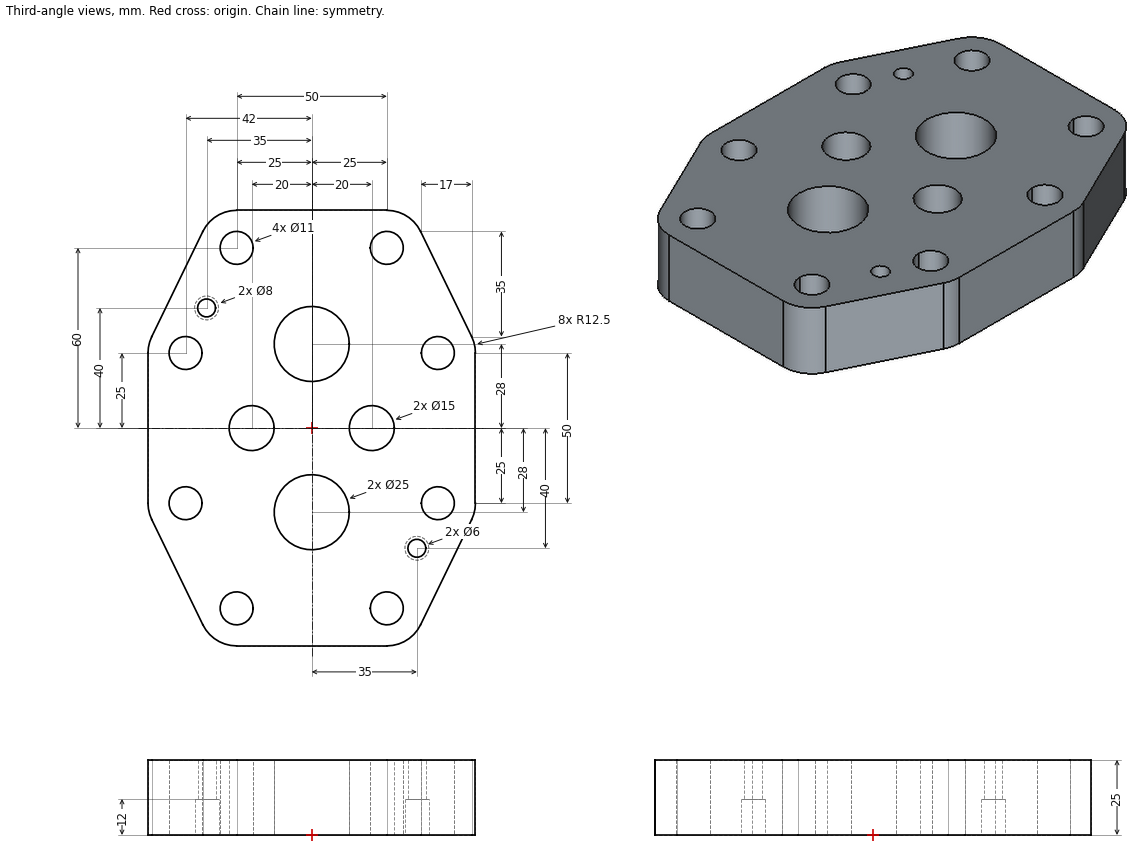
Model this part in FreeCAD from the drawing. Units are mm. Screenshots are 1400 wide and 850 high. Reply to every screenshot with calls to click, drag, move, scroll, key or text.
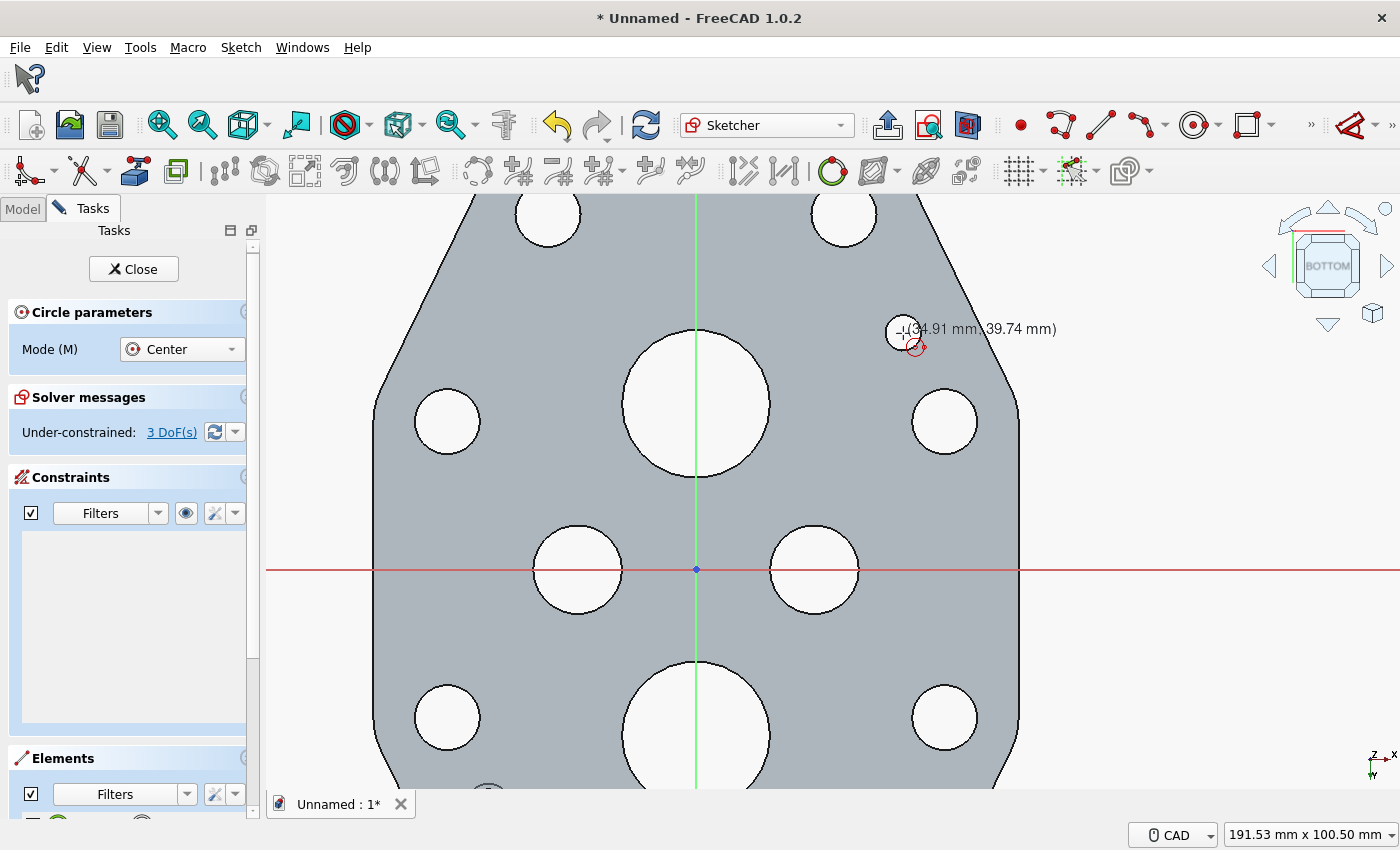
click(903, 333)
click(920, 316)
key(Escape)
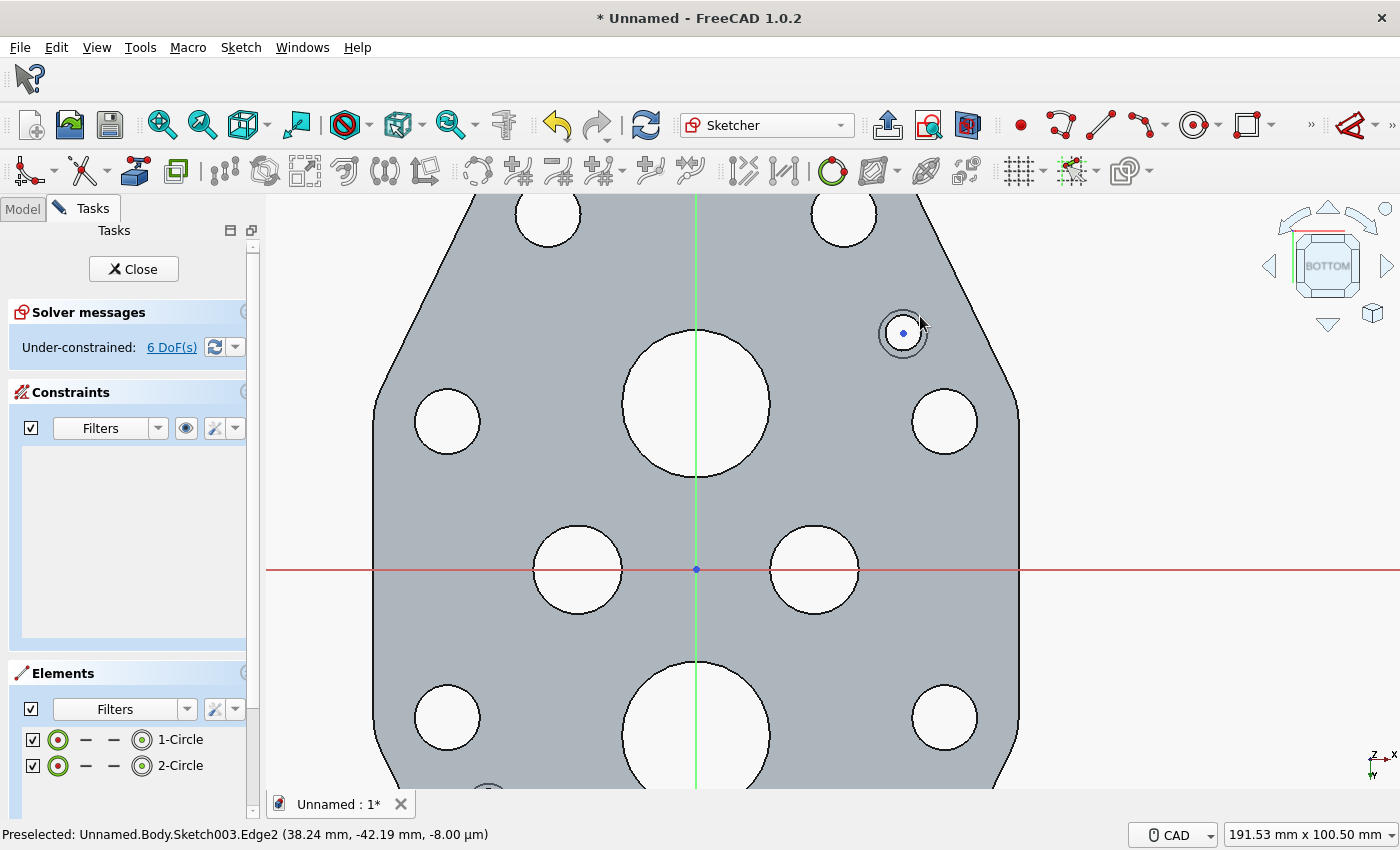
scroll(904, 333, down, 2)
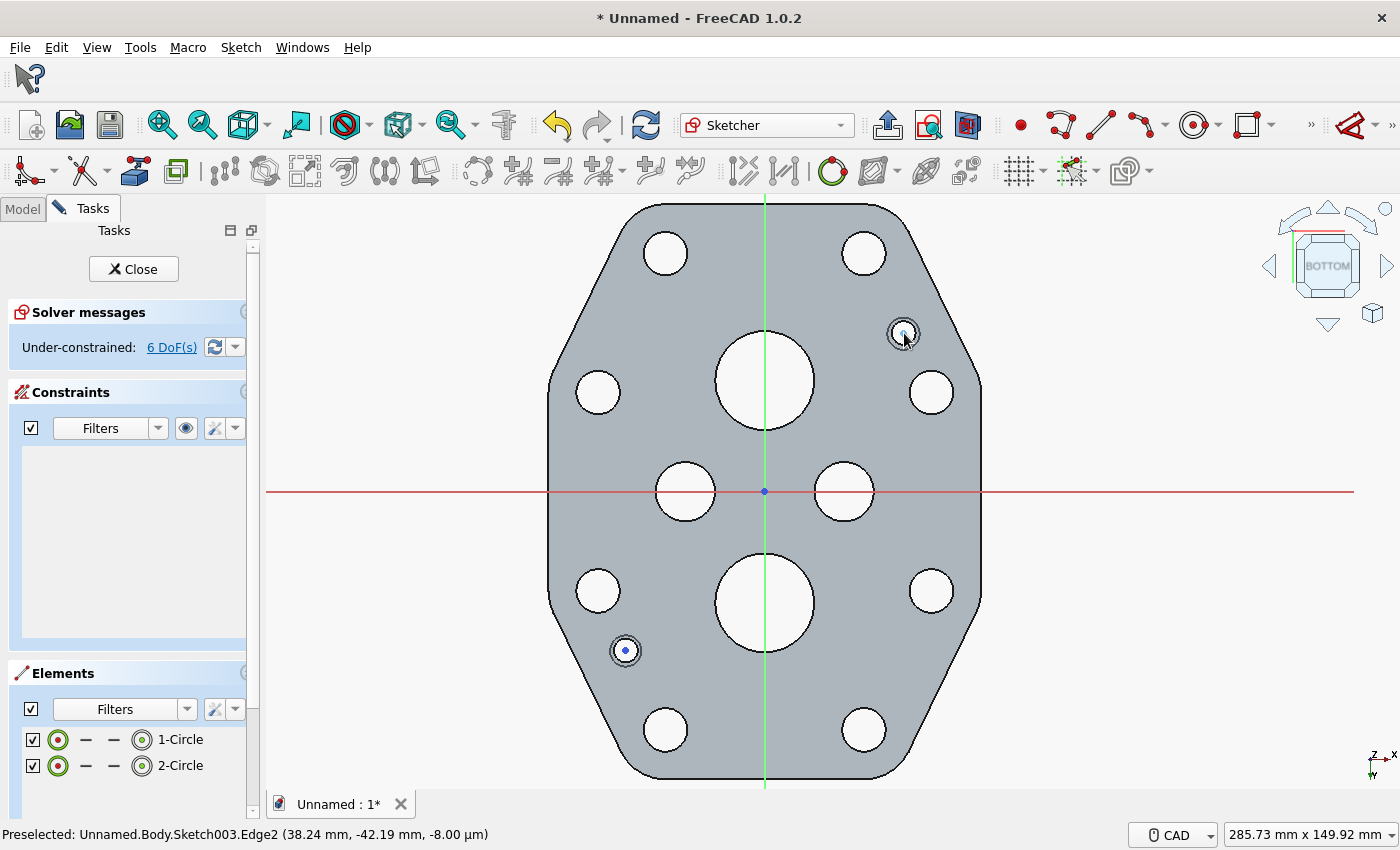
click(637, 640)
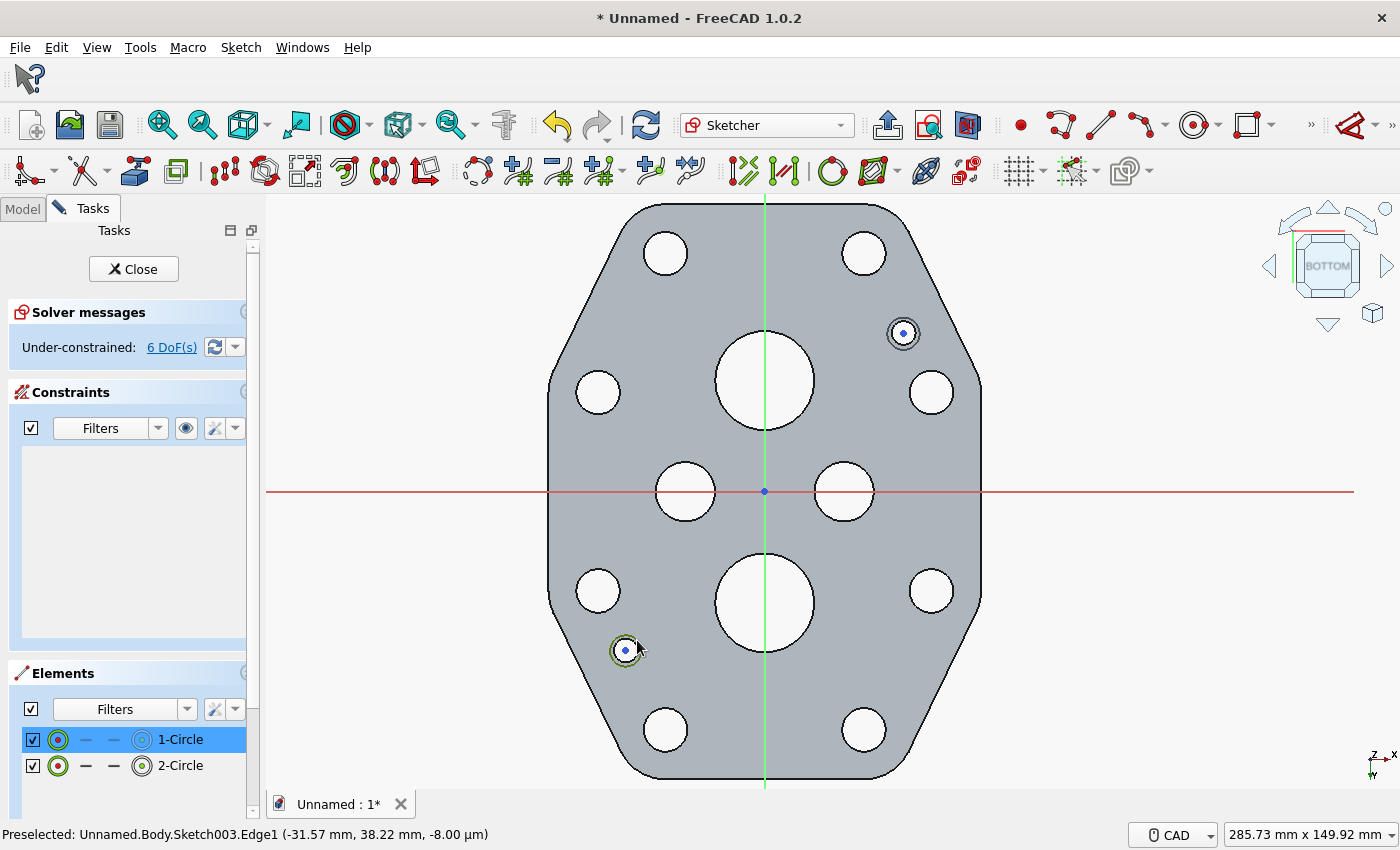
click(915, 322)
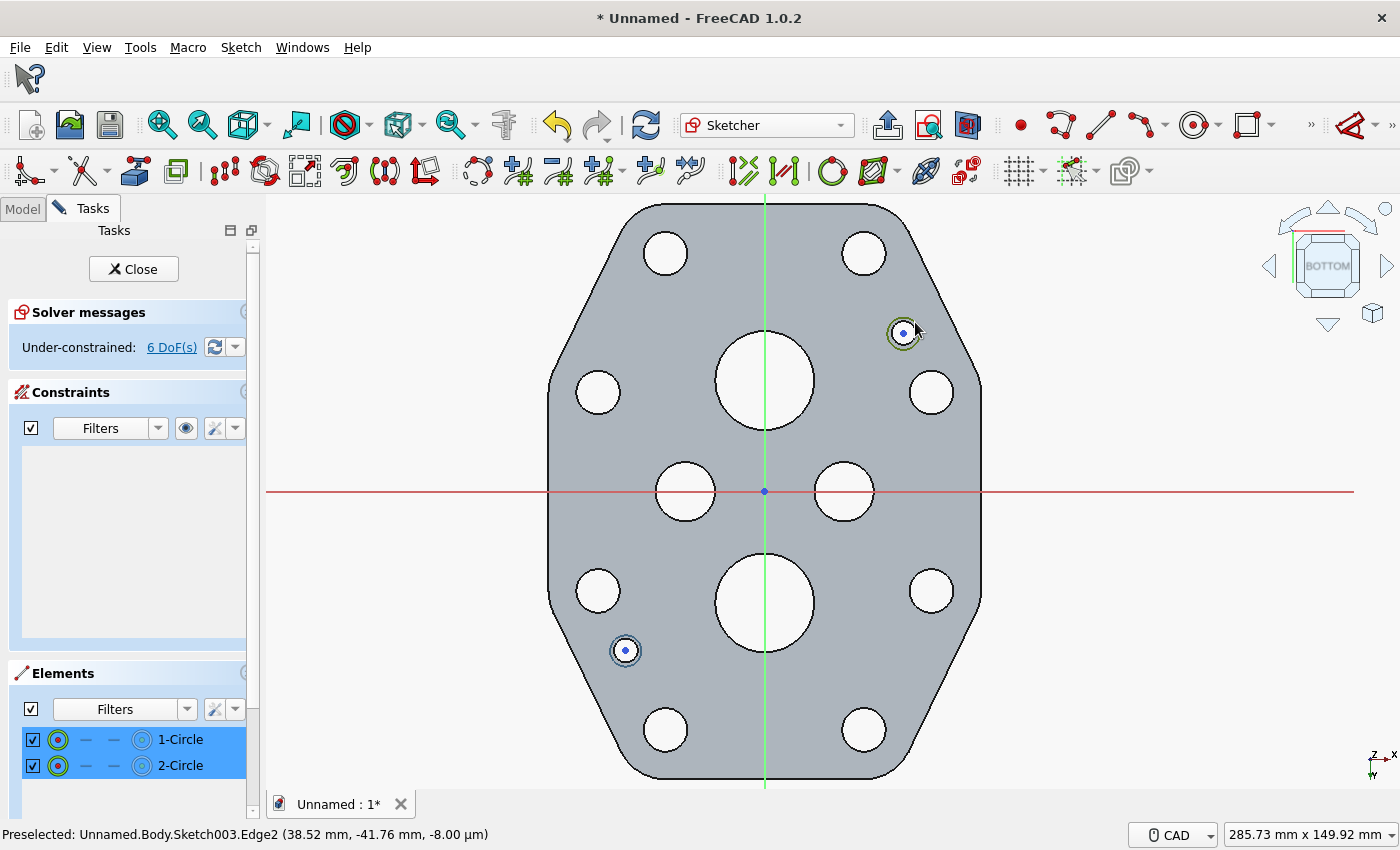
key(e)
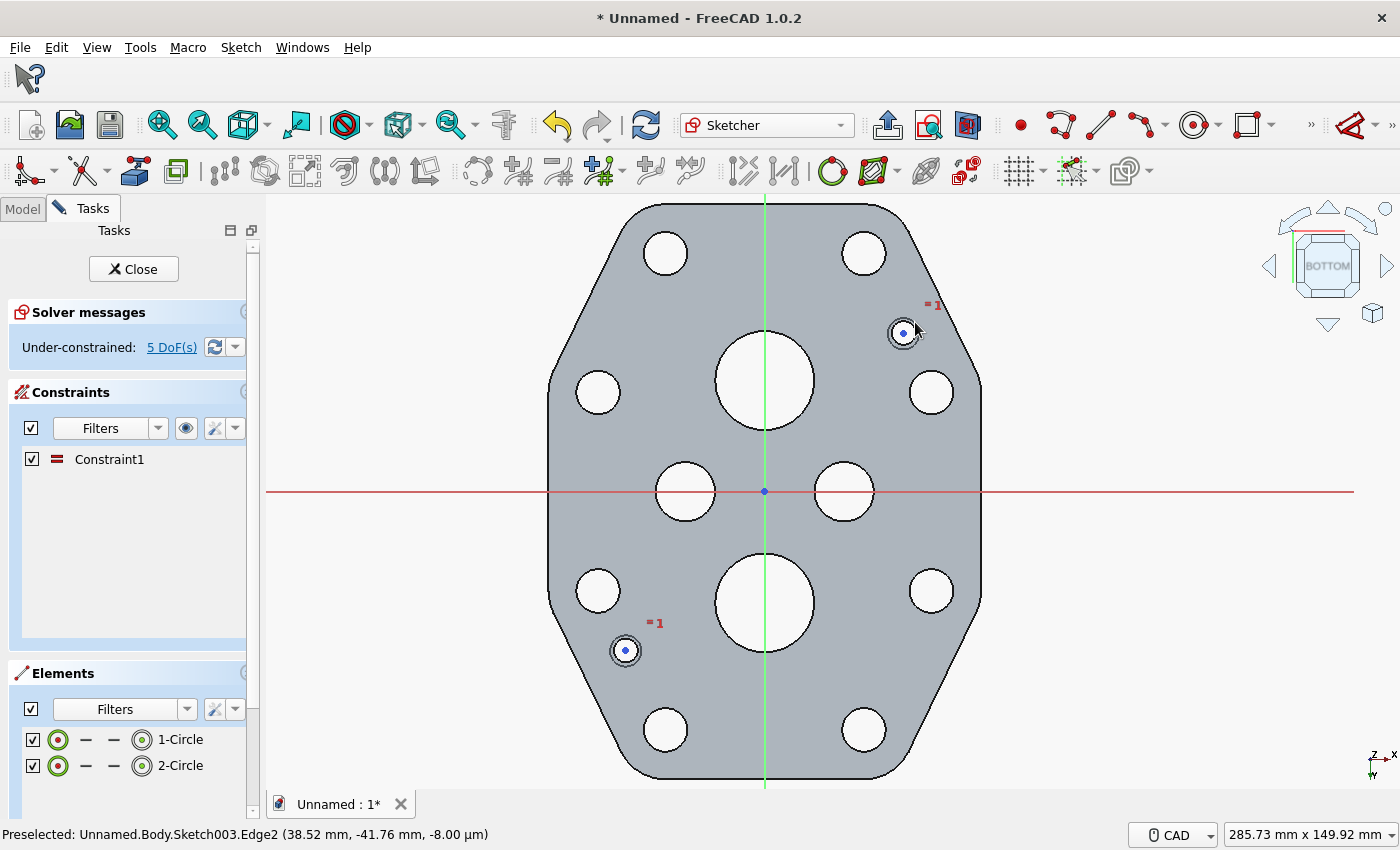
key(d)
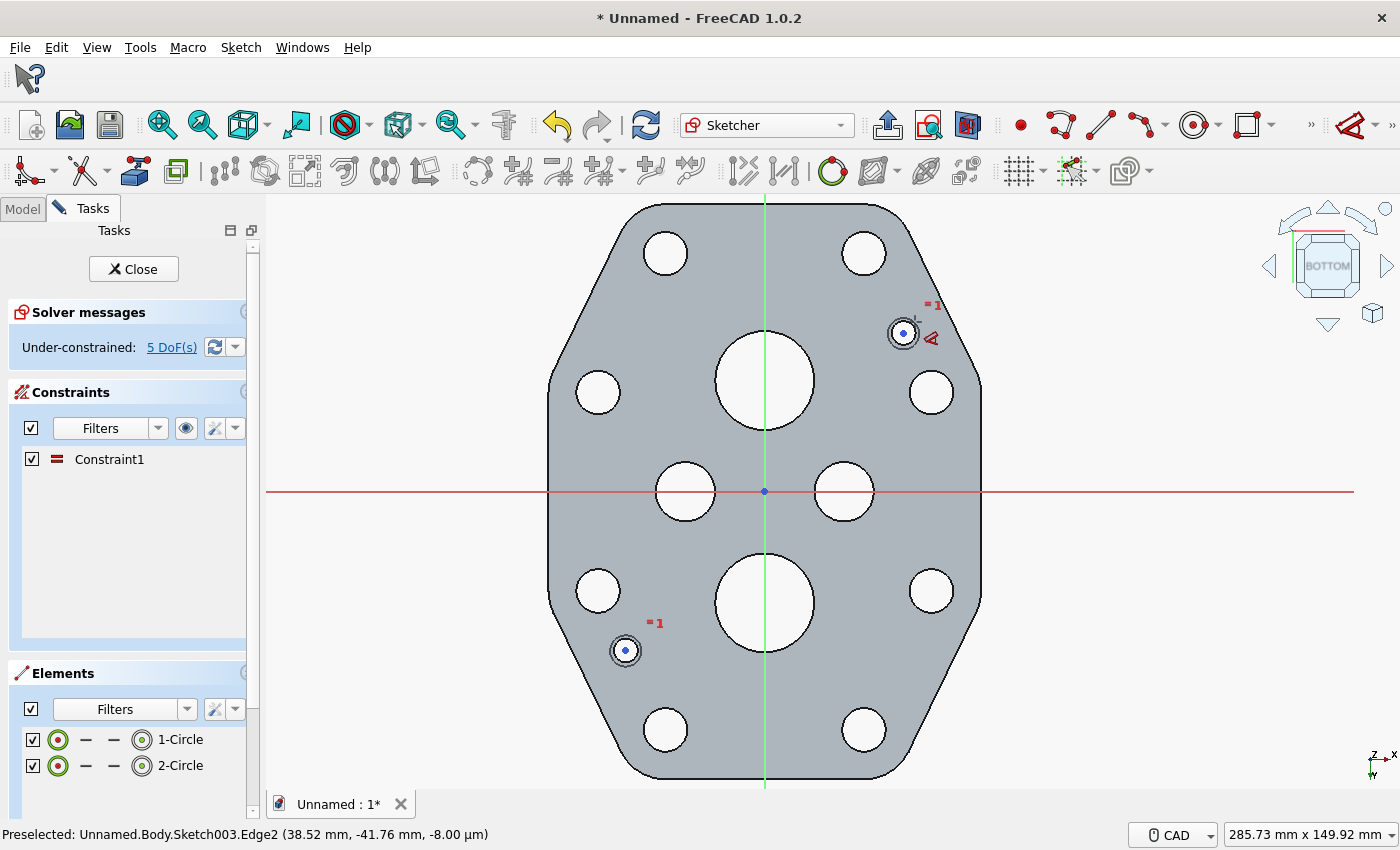
scroll(637, 640, up, 2)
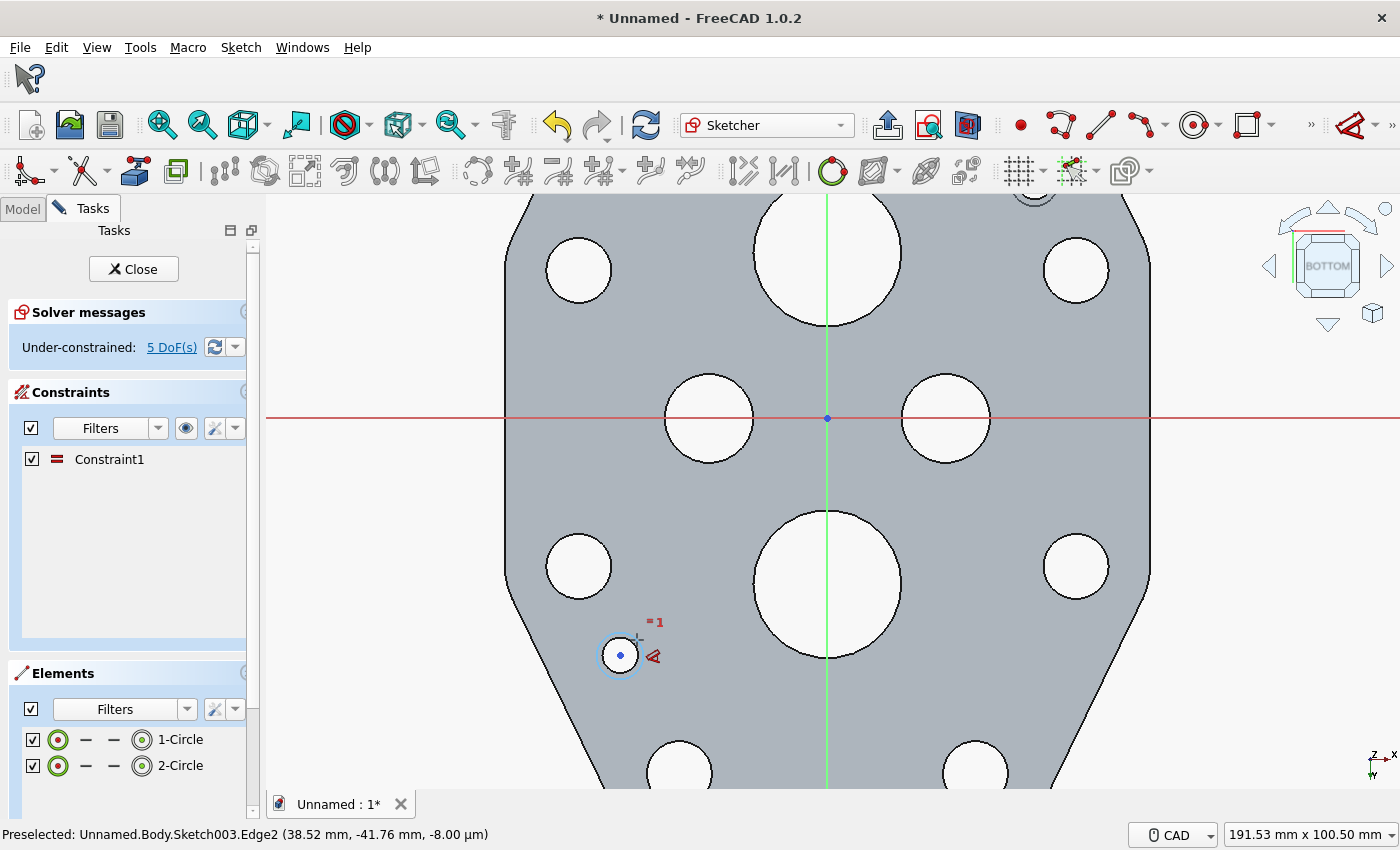
click(637, 639)
click(660, 616)